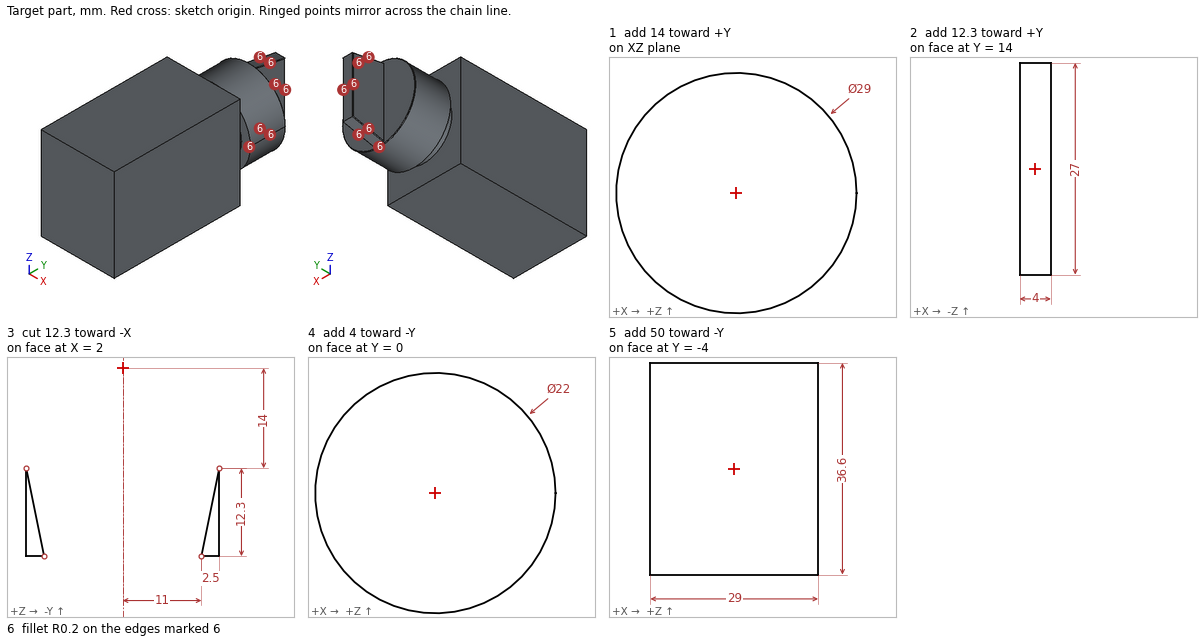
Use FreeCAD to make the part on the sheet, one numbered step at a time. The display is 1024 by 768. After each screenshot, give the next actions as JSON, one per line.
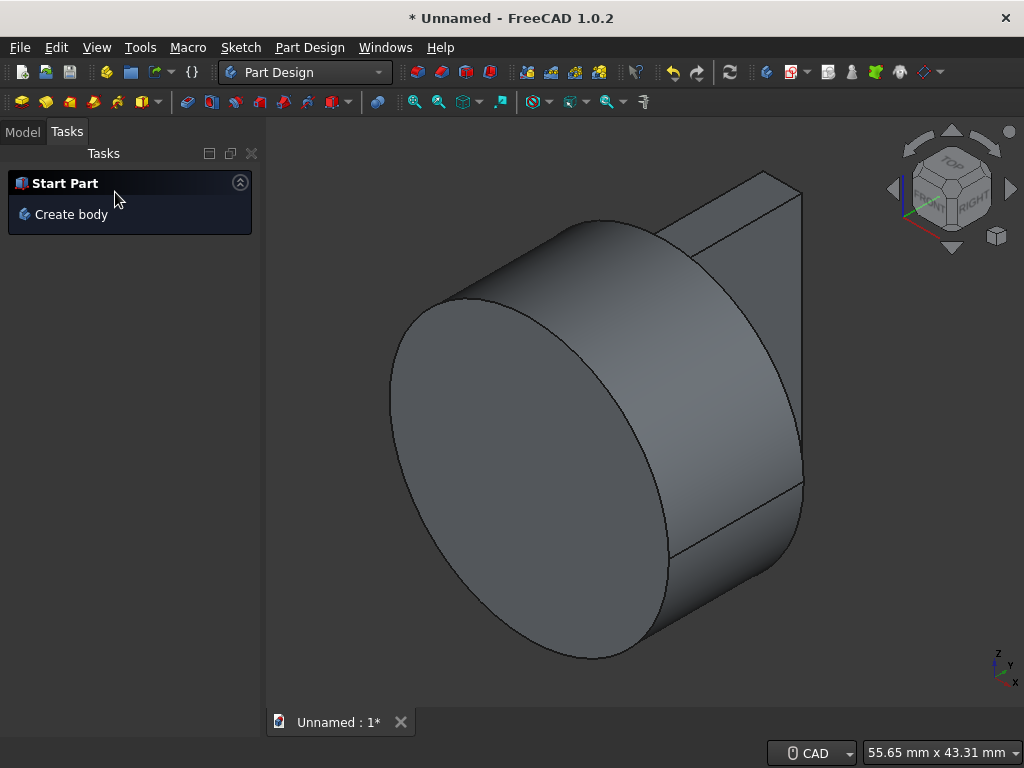
{"action": "left_click", "coordinate": [416, 102]}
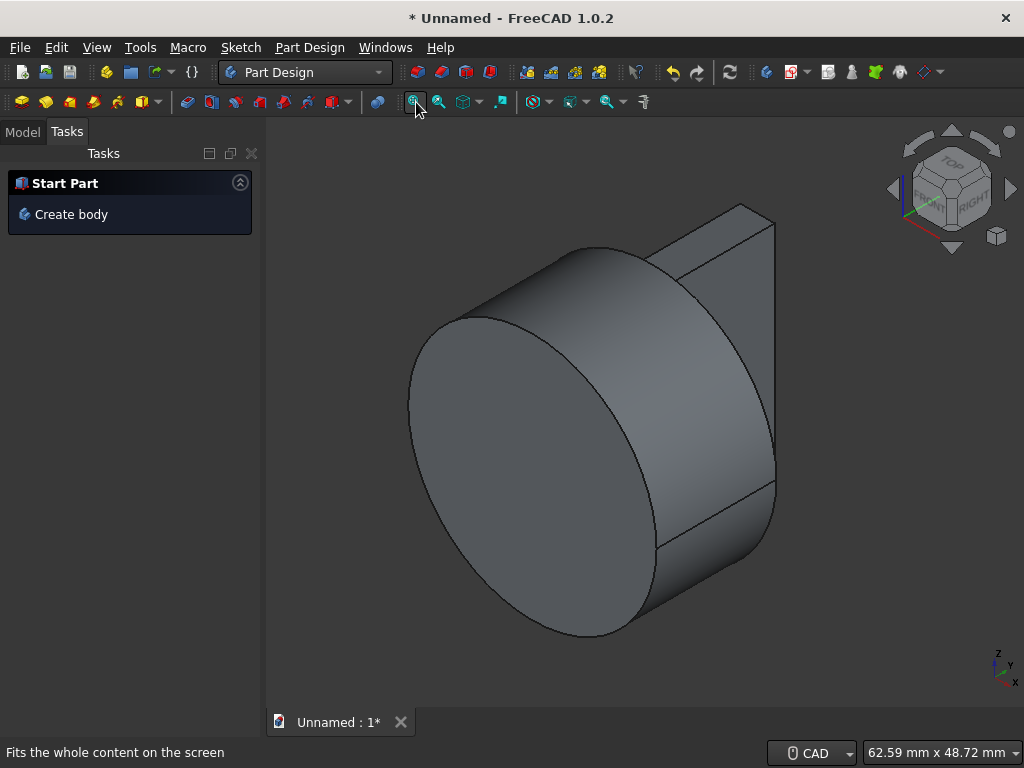
{"action": "left_click", "coordinate": [722, 310]}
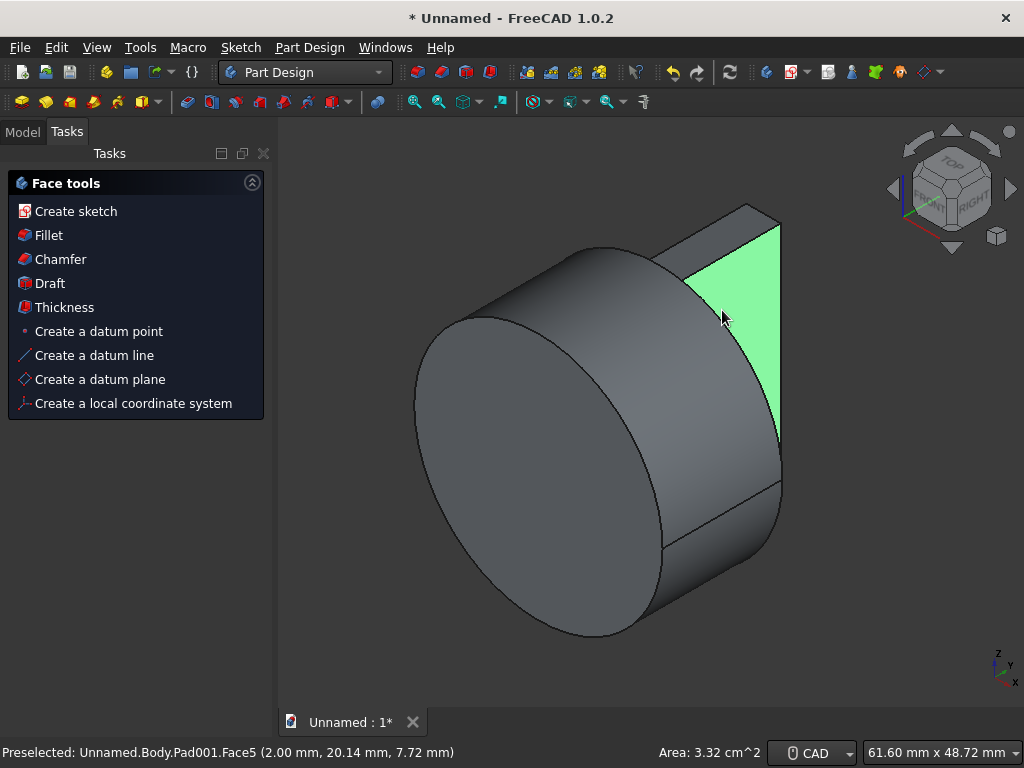
{"action": "left_click", "coordinate": [792, 72]}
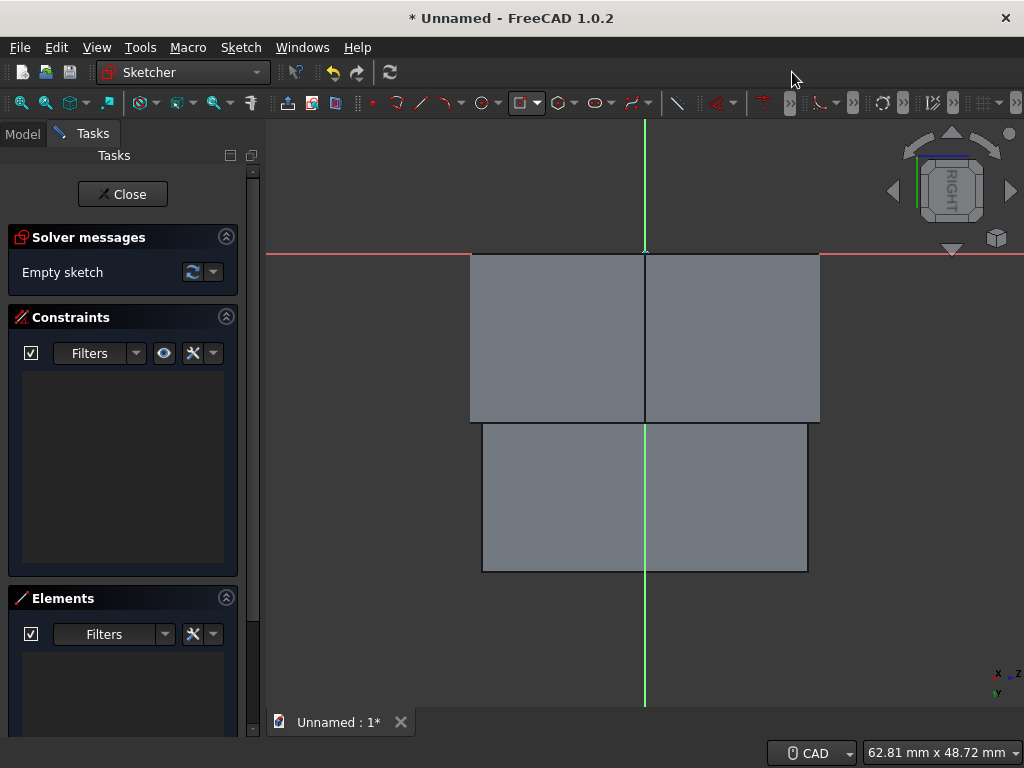
{"action": "key", "text": "g m"}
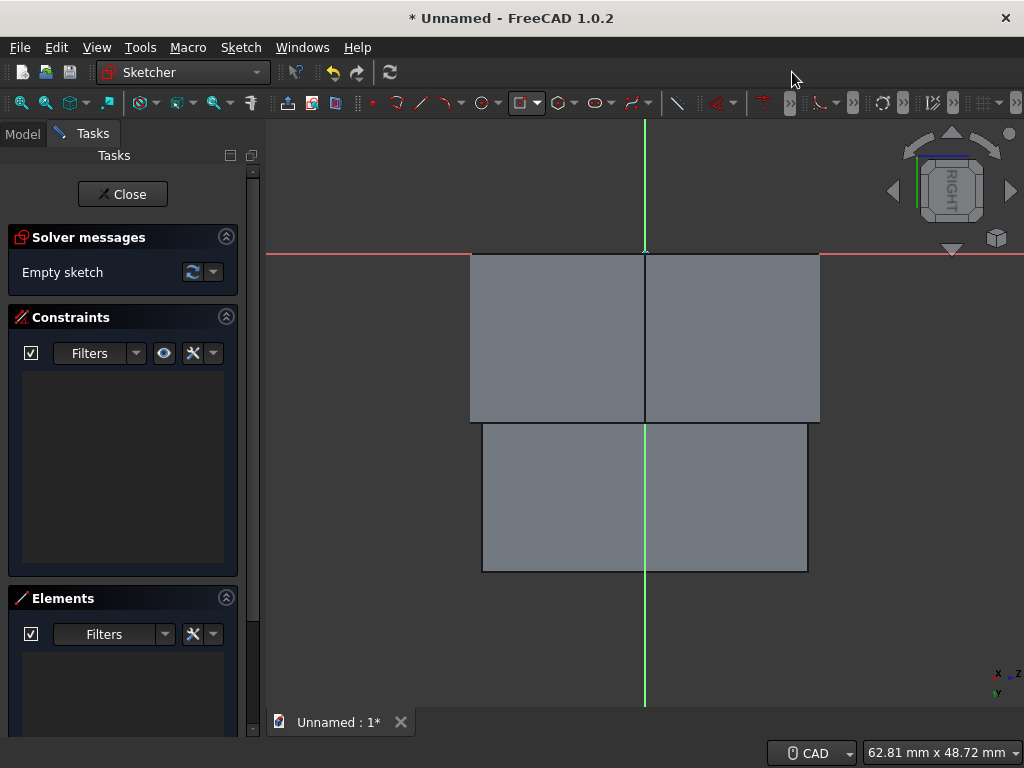
{"action": "left_click", "coordinate": [808, 423]}
{"action": "left_click", "coordinate": [778, 572]}
{"action": "left_click", "coordinate": [808, 572]}
{"action": "left_click", "coordinate": [808, 424]}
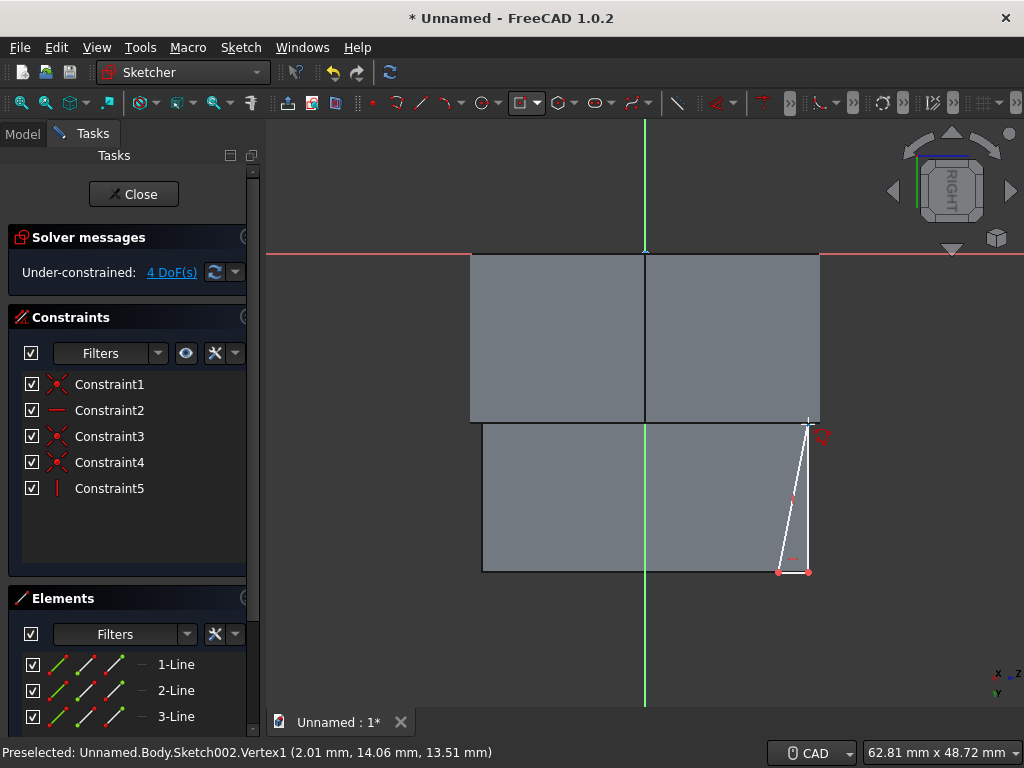
{"action": "left_click", "coordinate": [482, 423]}
{"action": "left_click", "coordinate": [482, 572]}
{"action": "left_click", "coordinate": [512, 572]}
{"action": "left_click", "coordinate": [482, 424]}
{"action": "key", "text": "Escape"}
{"action": "key", "text": "Escape"}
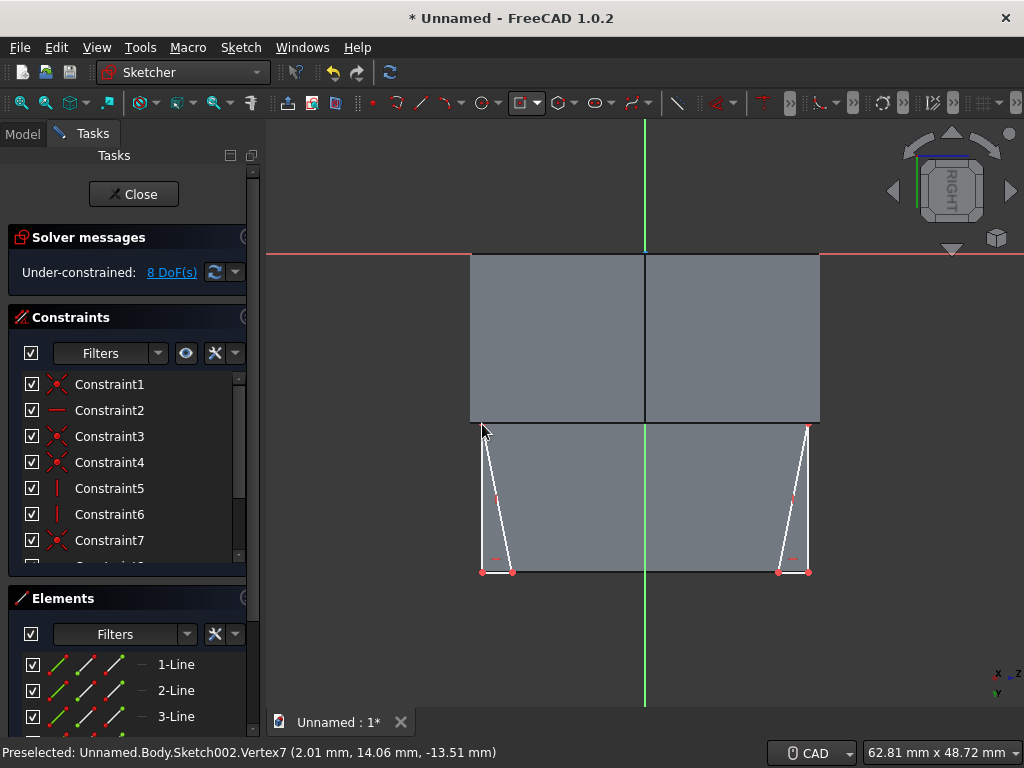
{"action": "left_click", "coordinate": [808, 424]}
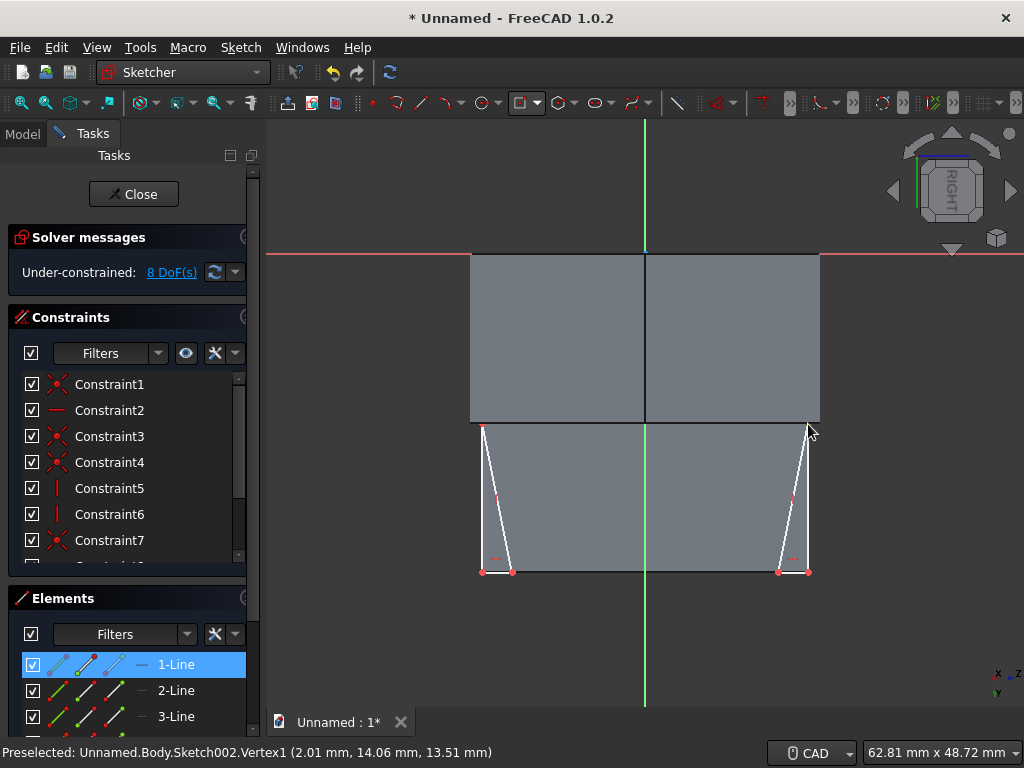
{"action": "left_click", "coordinate": [482, 424]}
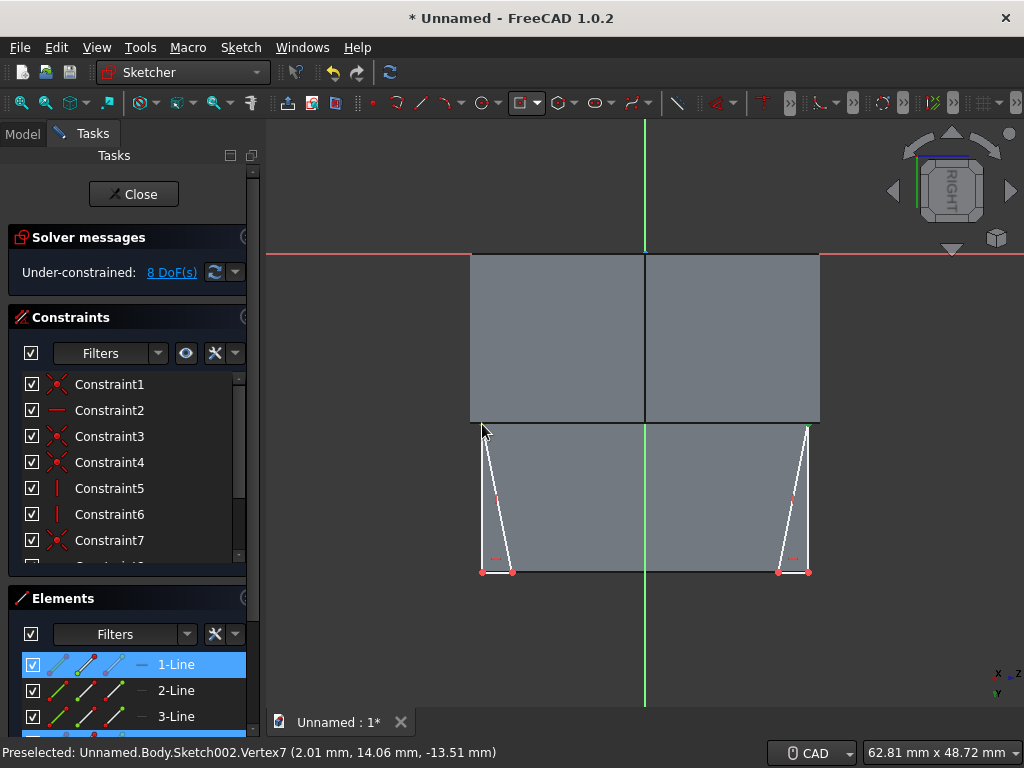
{"action": "left_click", "coordinate": [645, 641]}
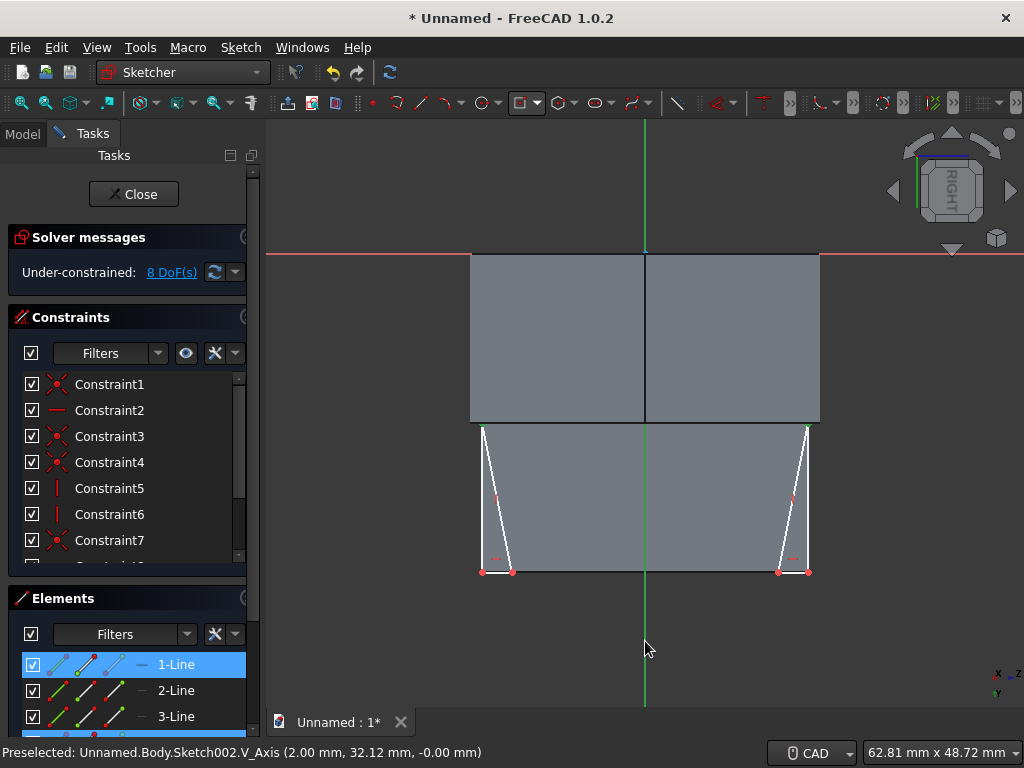
{"action": "key", "text": "s"}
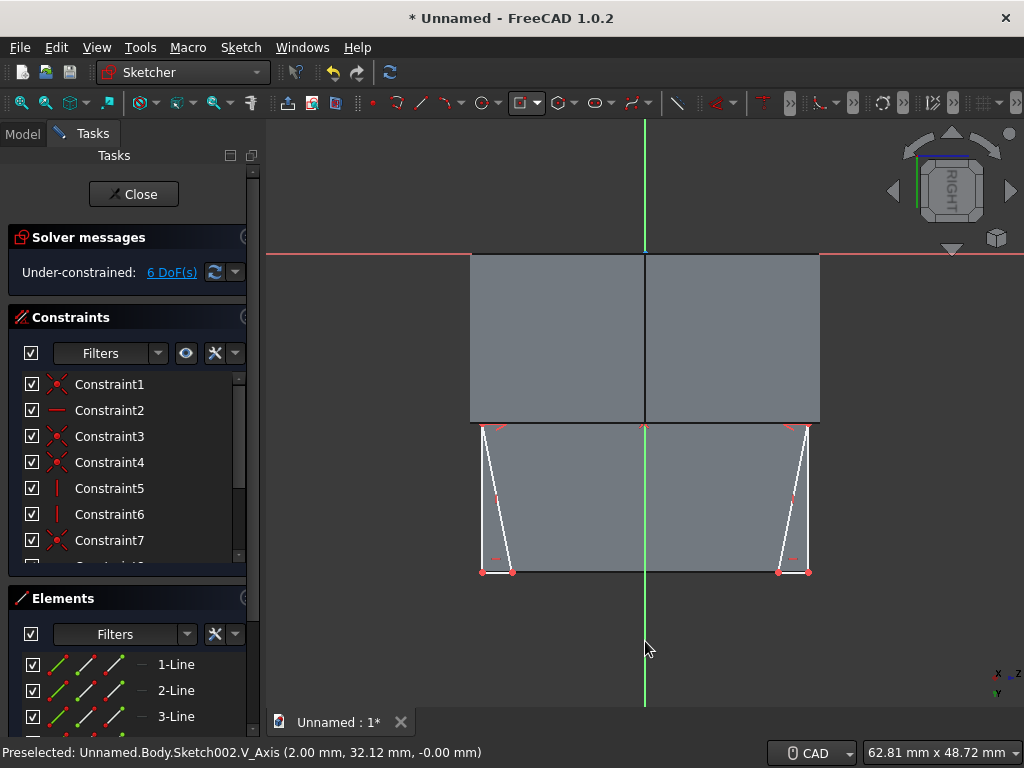
{"action": "left_click", "coordinate": [778, 573]}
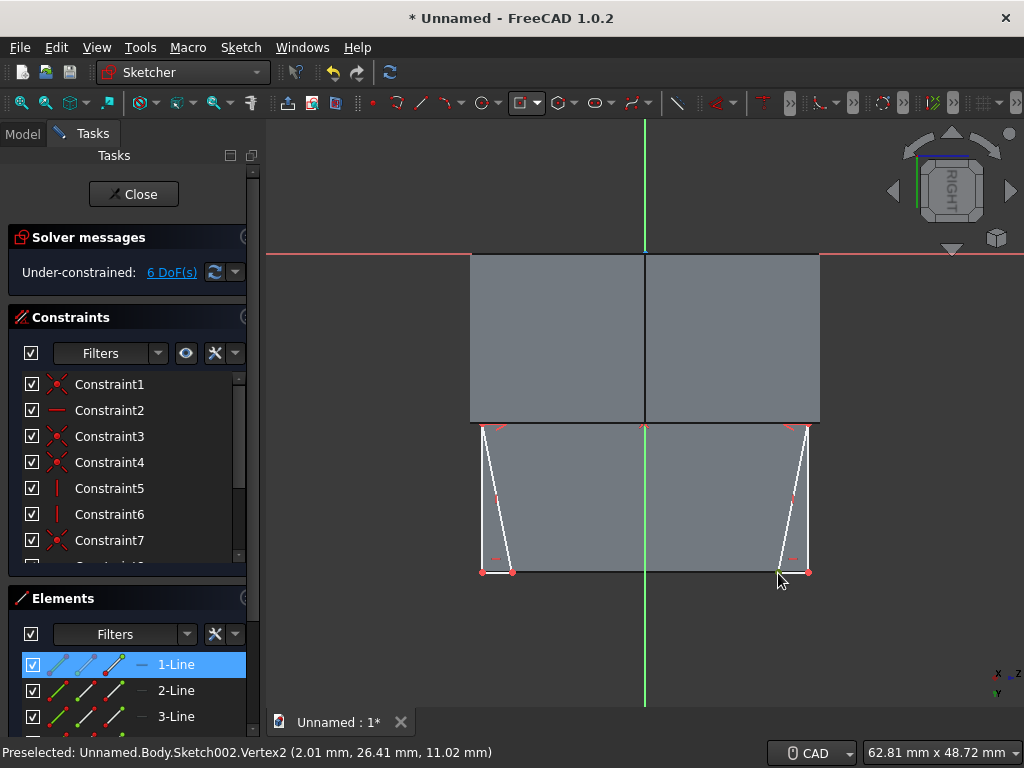
{"action": "left_click", "coordinate": [512, 573]}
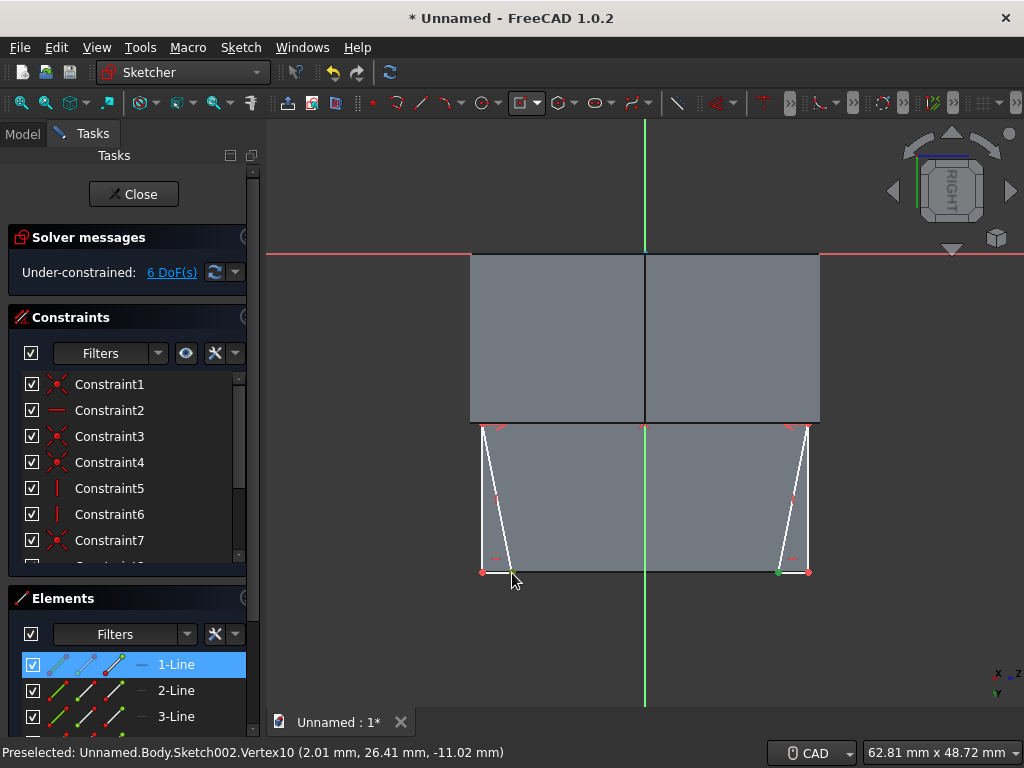
{"action": "left_click", "coordinate": [645, 641]}